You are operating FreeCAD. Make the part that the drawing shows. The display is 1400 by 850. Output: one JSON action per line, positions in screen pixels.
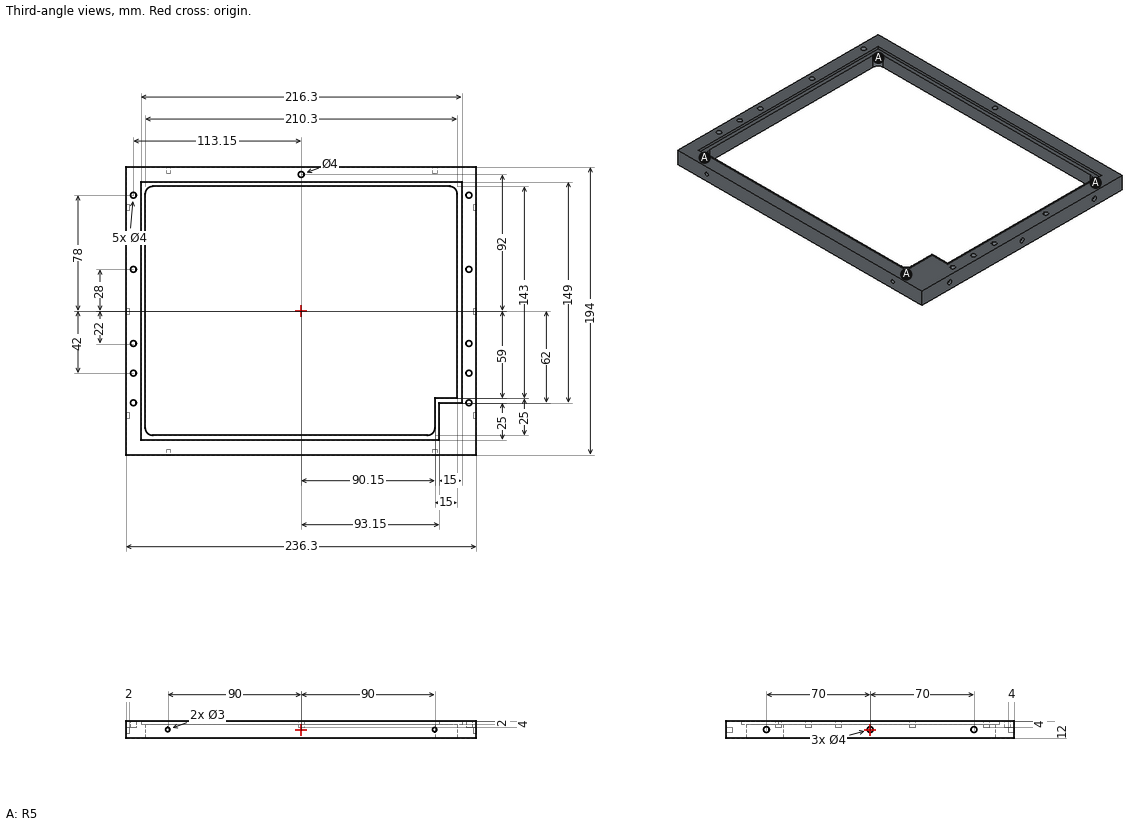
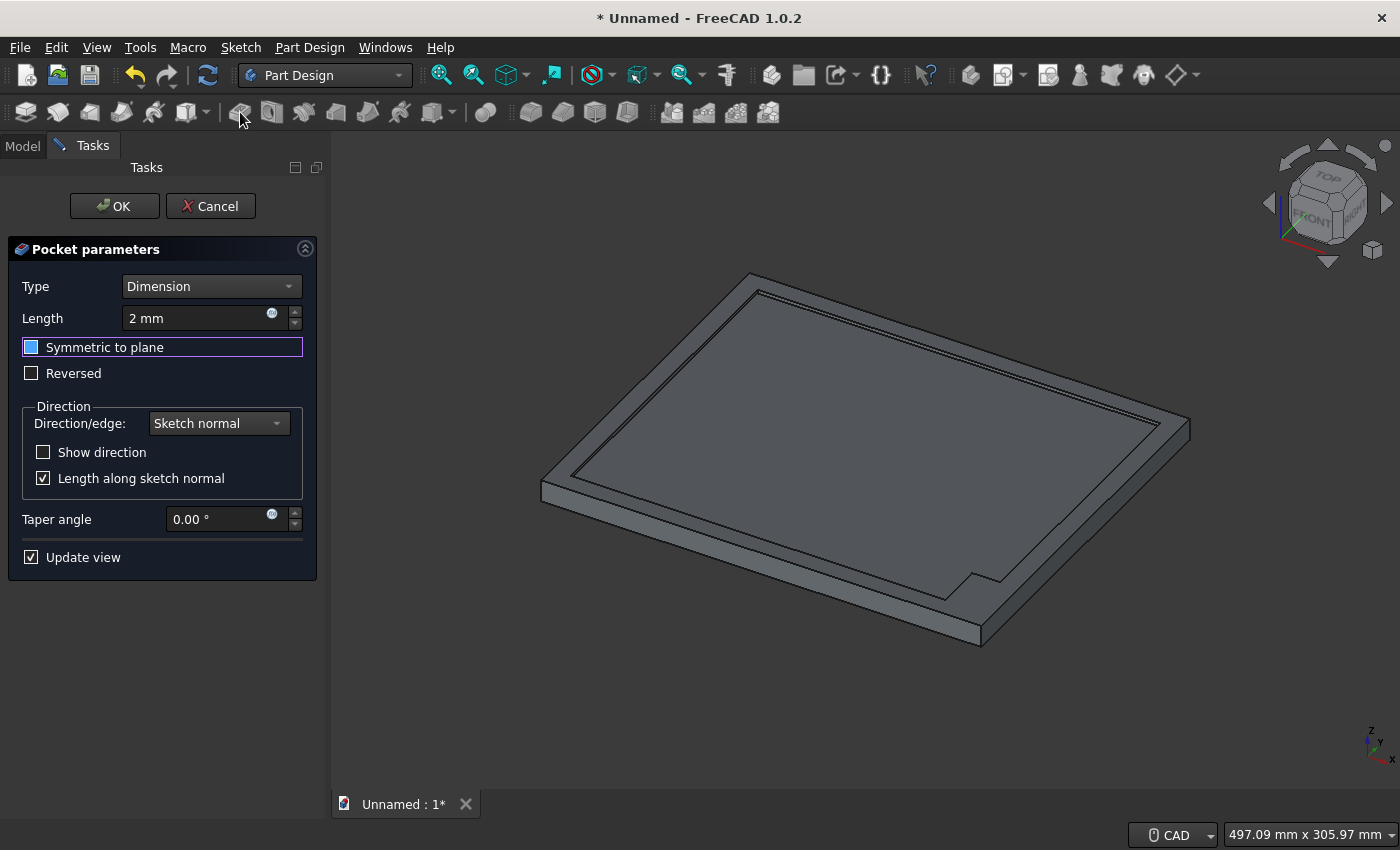
{"action": "left_click", "coordinate": [115, 206]}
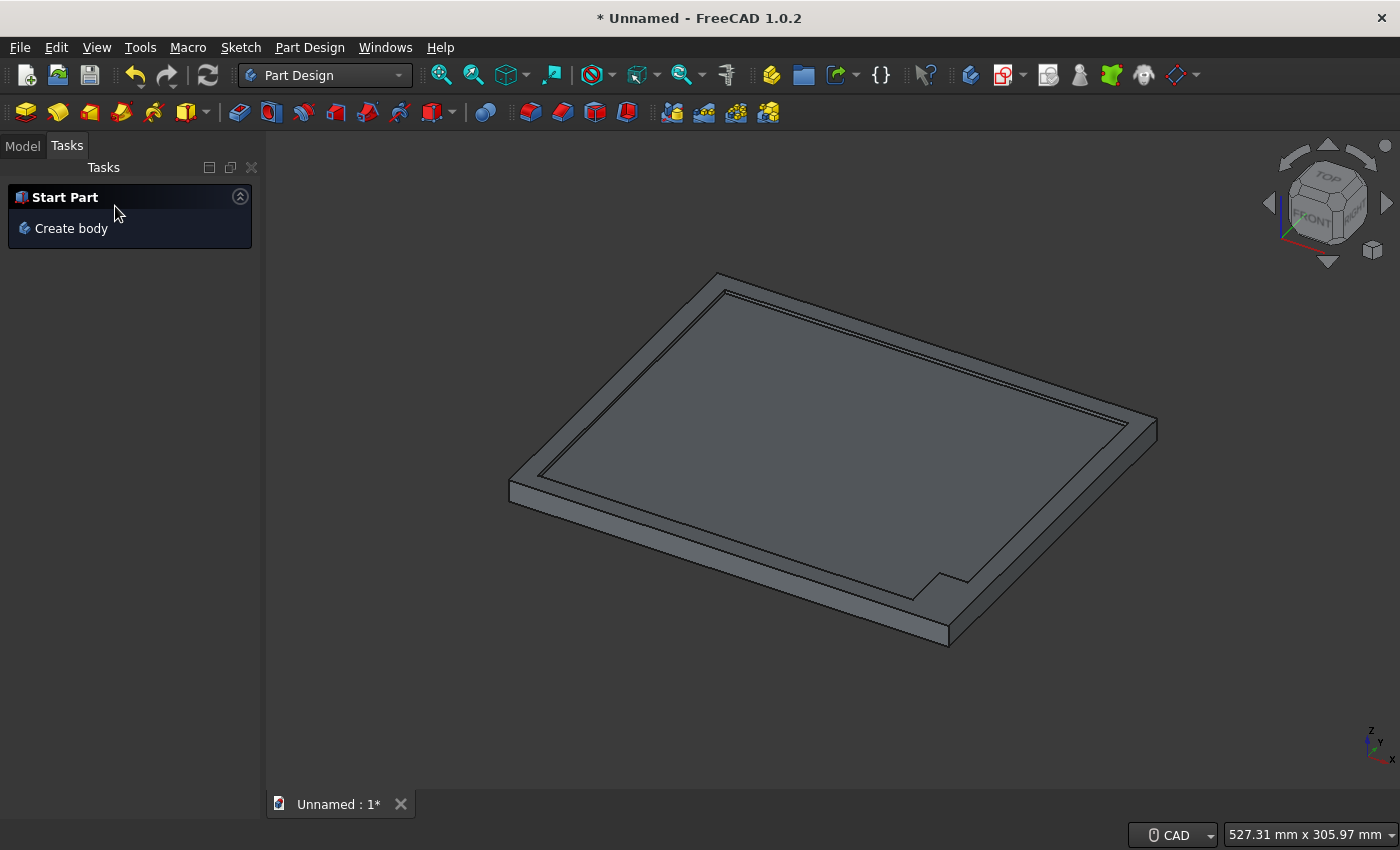
{"action": "left_click", "coordinate": [833, 452]}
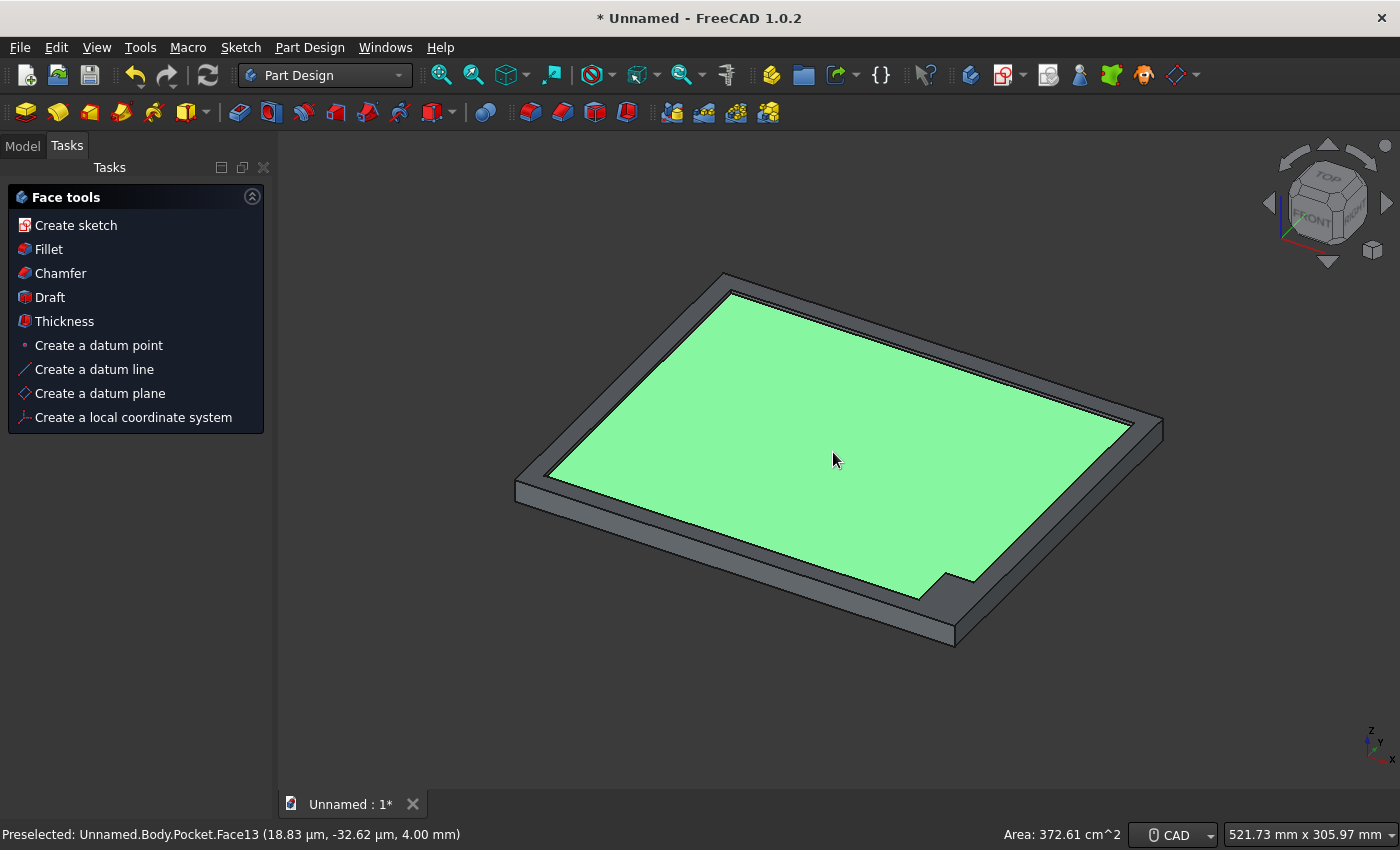
{"action": "left_click", "coordinate": [1004, 76]}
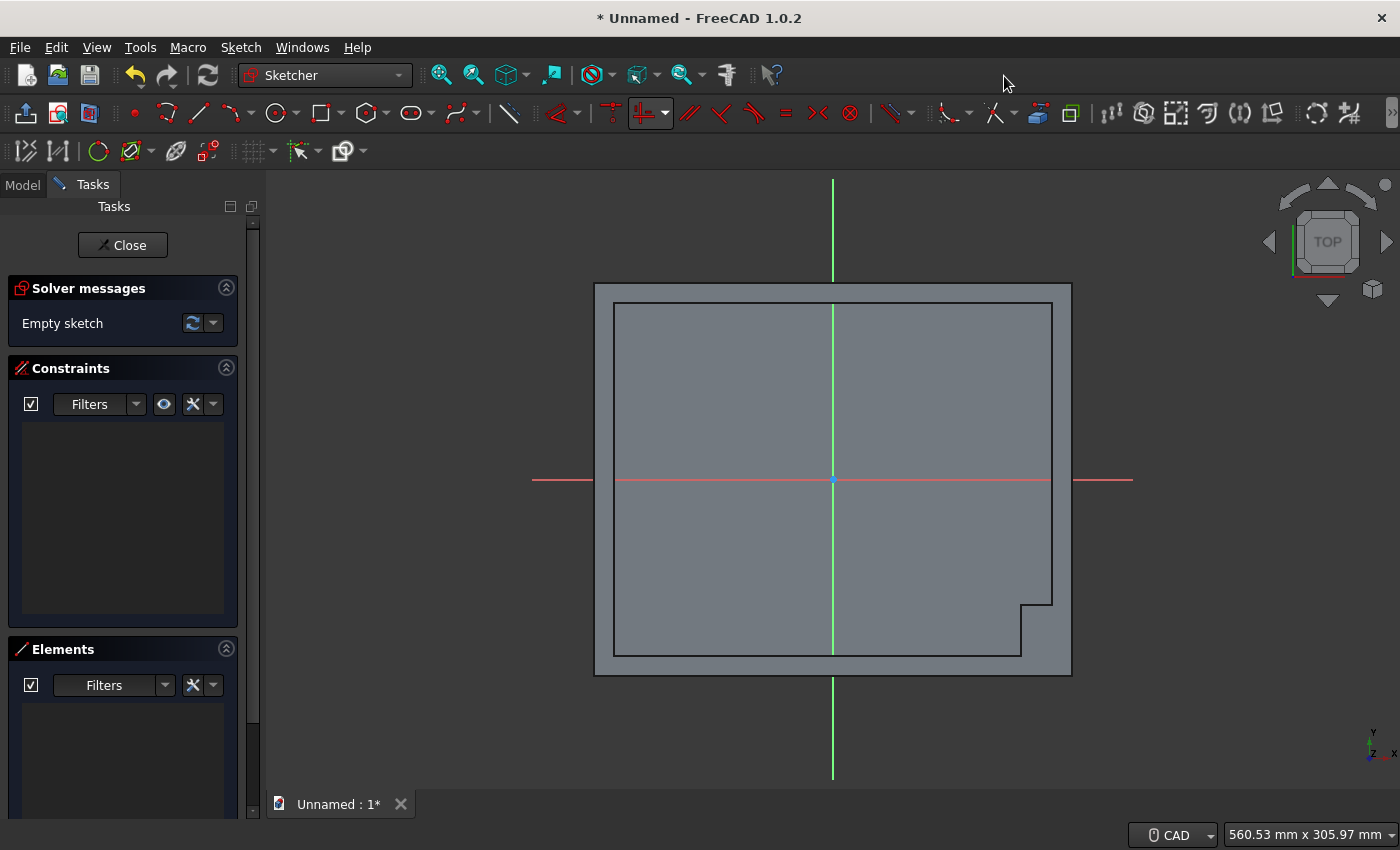
{"action": "left_click", "coordinate": [168, 114]}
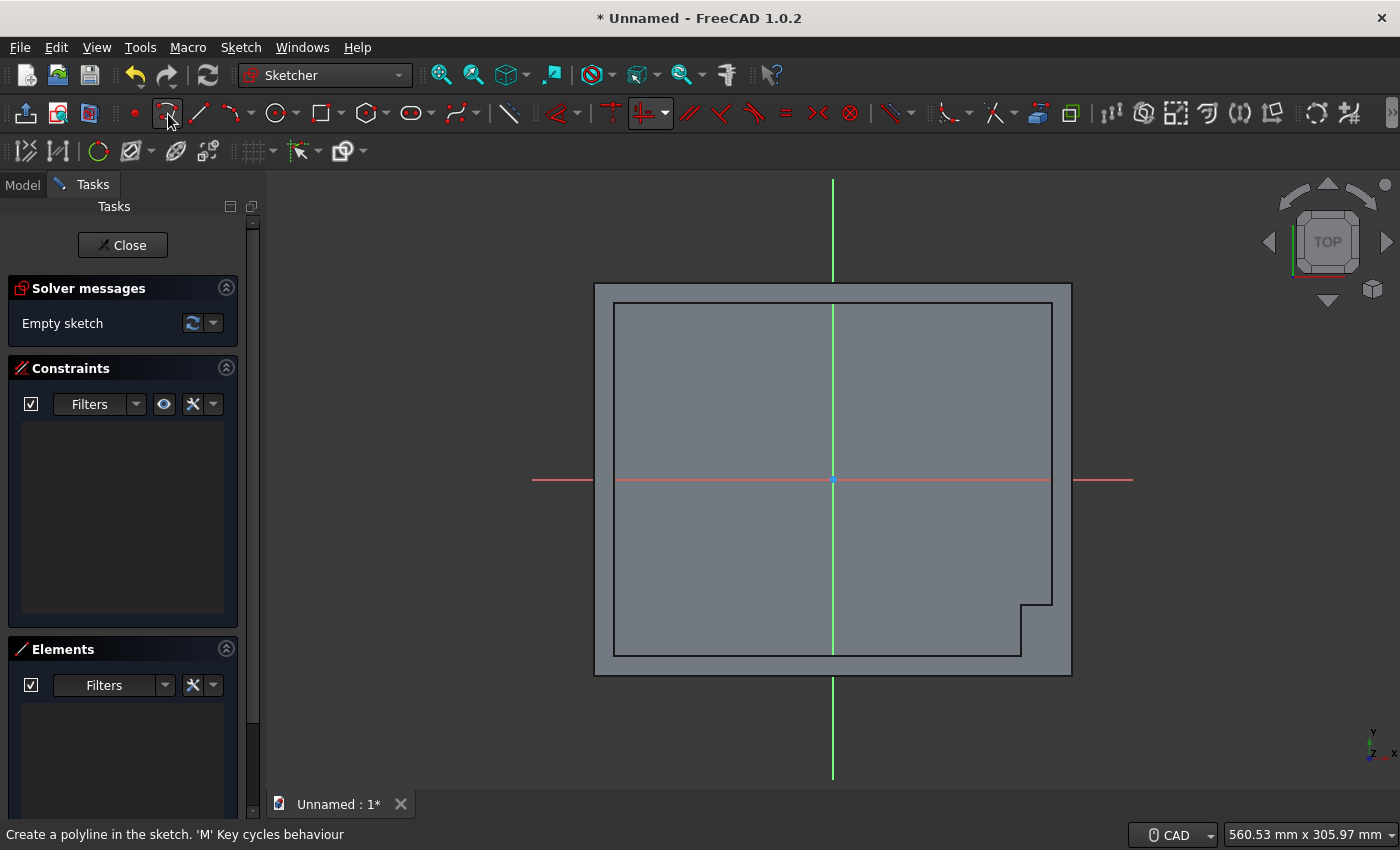
{"action": "left_click", "coordinate": [1015, 599]}
{"action": "left_click", "coordinate": [1046, 599]}
{"action": "left_click", "coordinate": [1046, 310]}
{"action": "left_click", "coordinate": [620, 310]}
{"action": "left_click", "coordinate": [620, 649]}
{"action": "left_click", "coordinate": [1015, 649]}
{"action": "left_click", "coordinate": [1015, 600]}
{"action": "key", "text": "Escape"}
{"action": "key", "text": "Escape"}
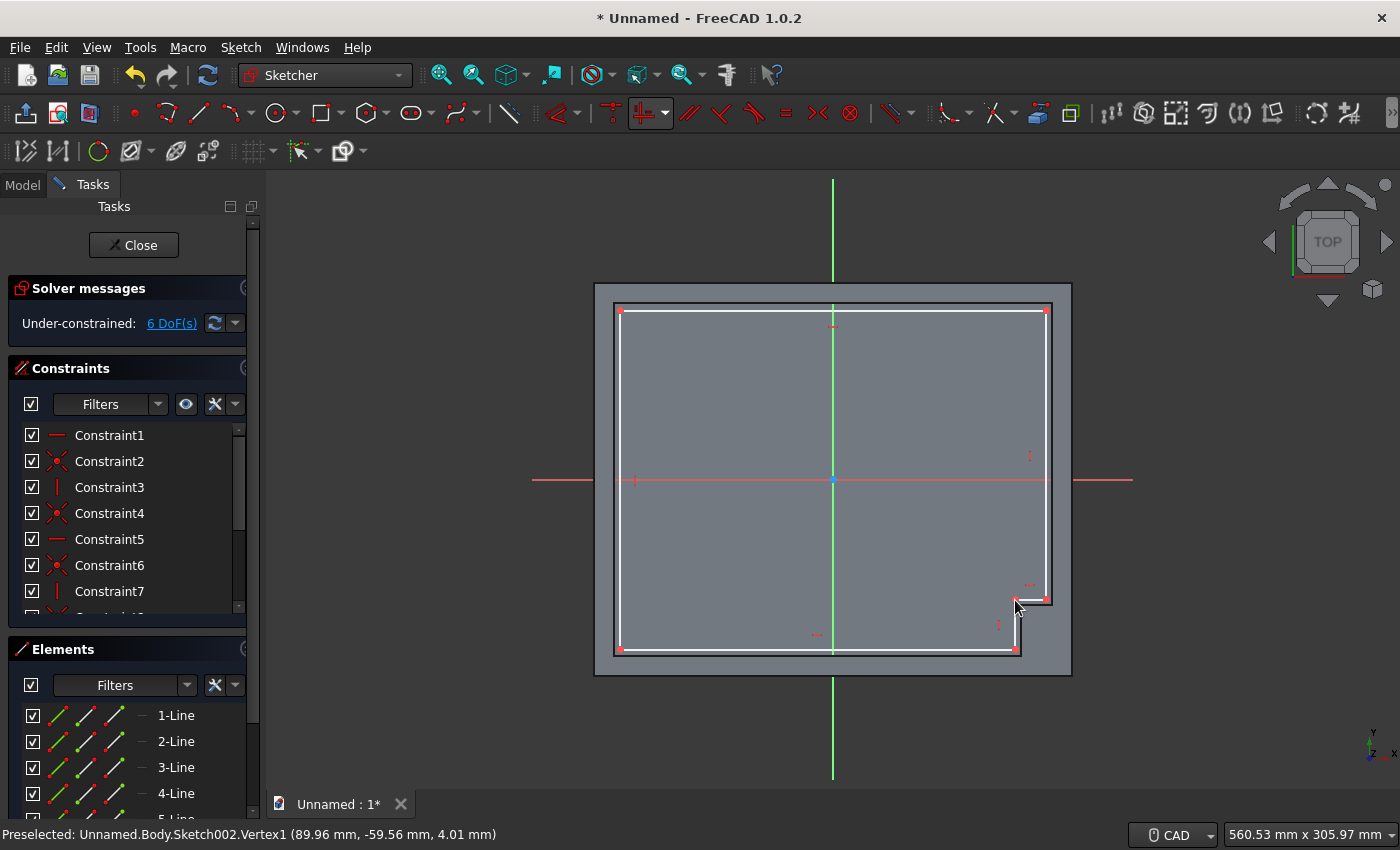
{"action": "left_click", "coordinate": [556, 114]}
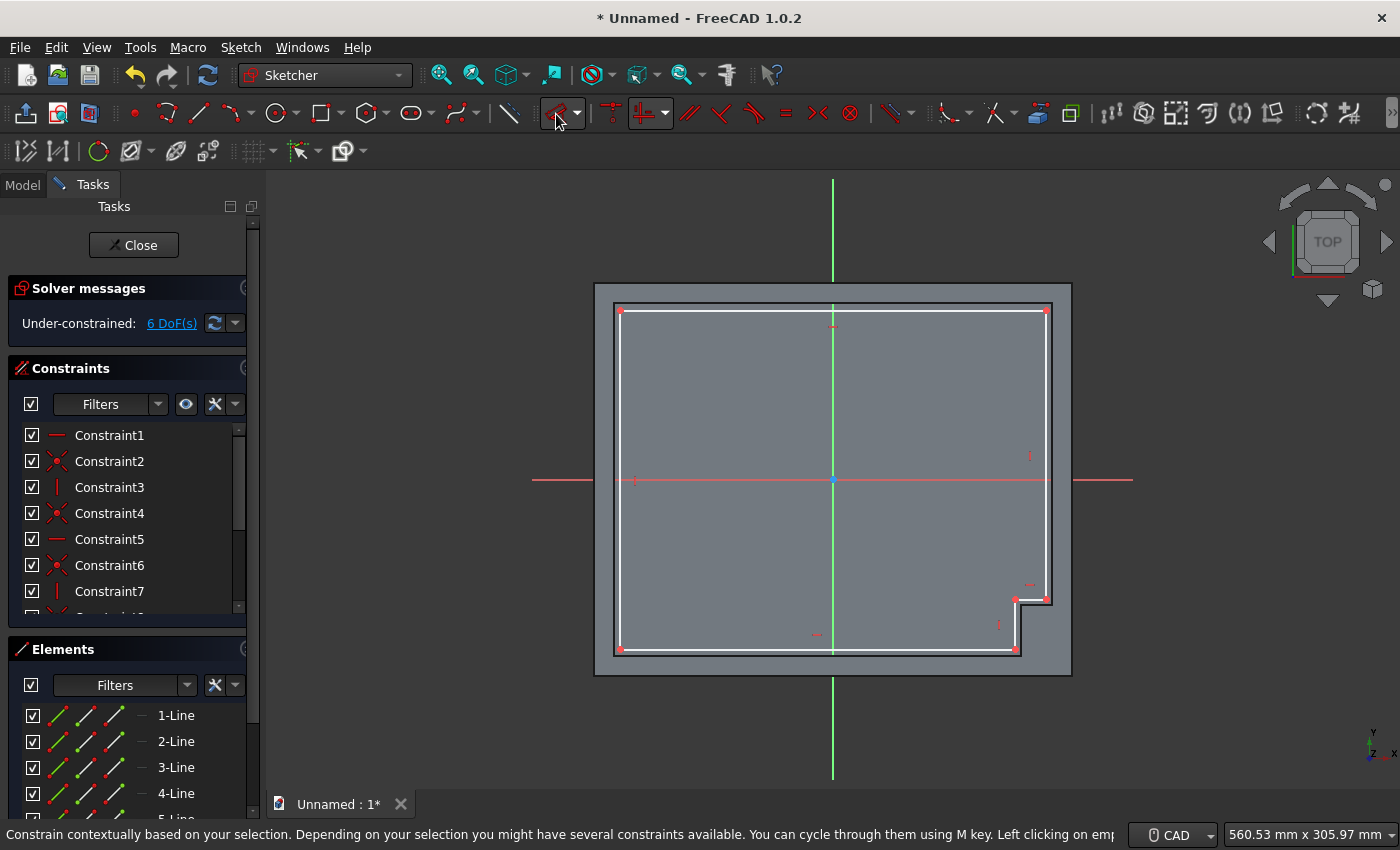
{"action": "scroll", "coordinate": [1024, 600], "scroll_direction": "up", "scroll_amount": 2}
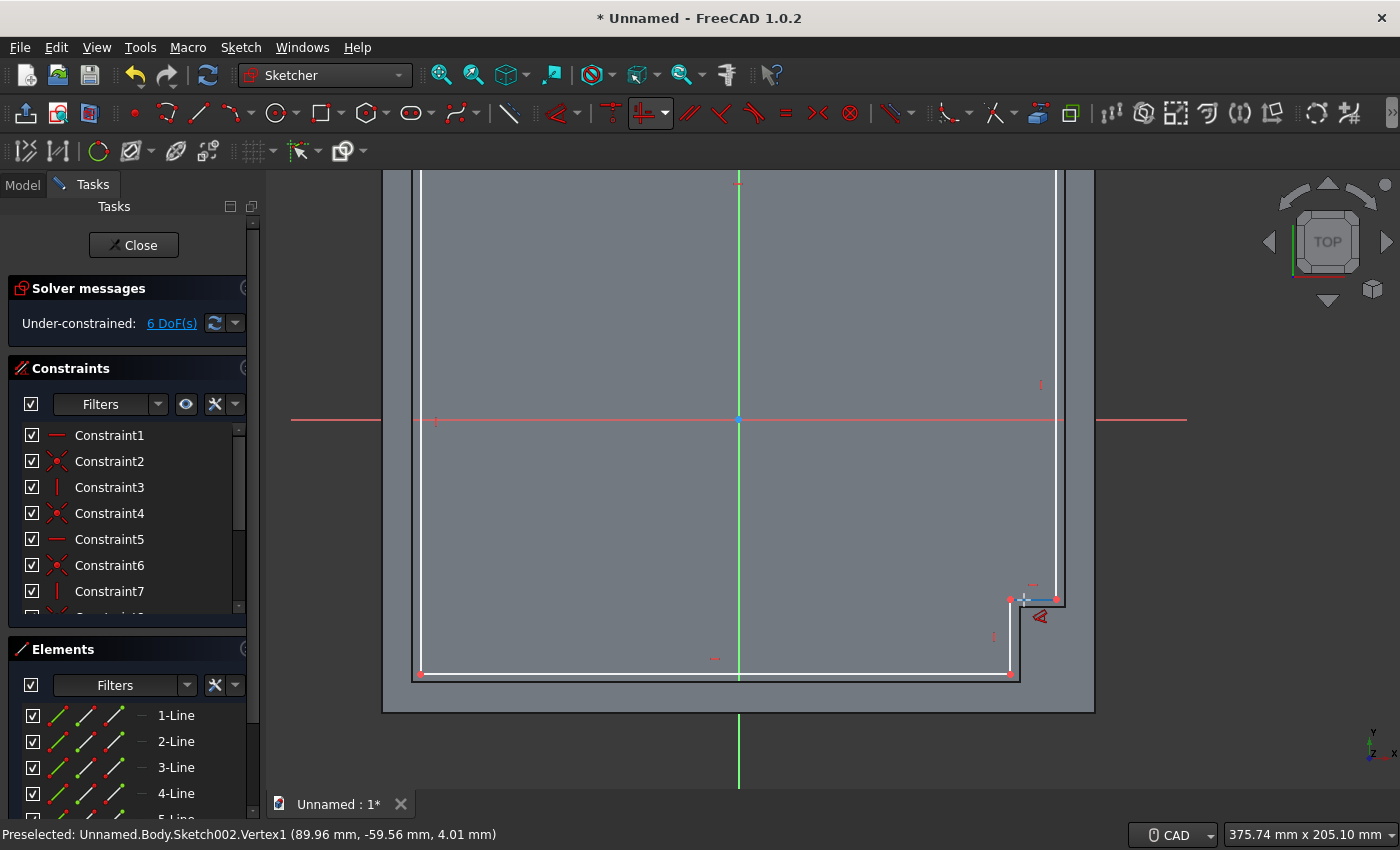
{"action": "left_click", "coordinate": [1024, 600]}
{"action": "left_click", "coordinate": [1033, 634]}